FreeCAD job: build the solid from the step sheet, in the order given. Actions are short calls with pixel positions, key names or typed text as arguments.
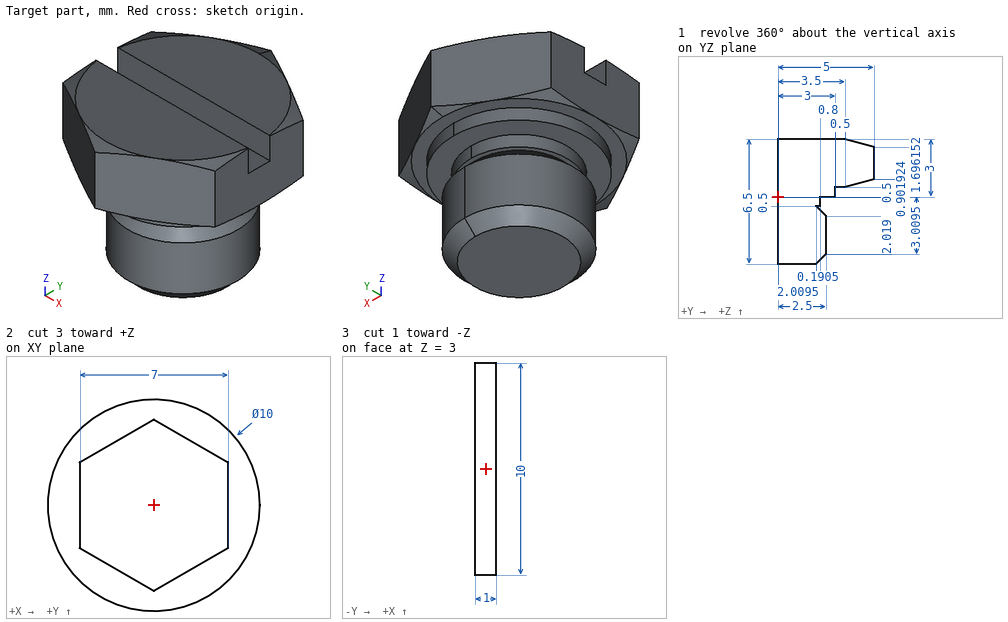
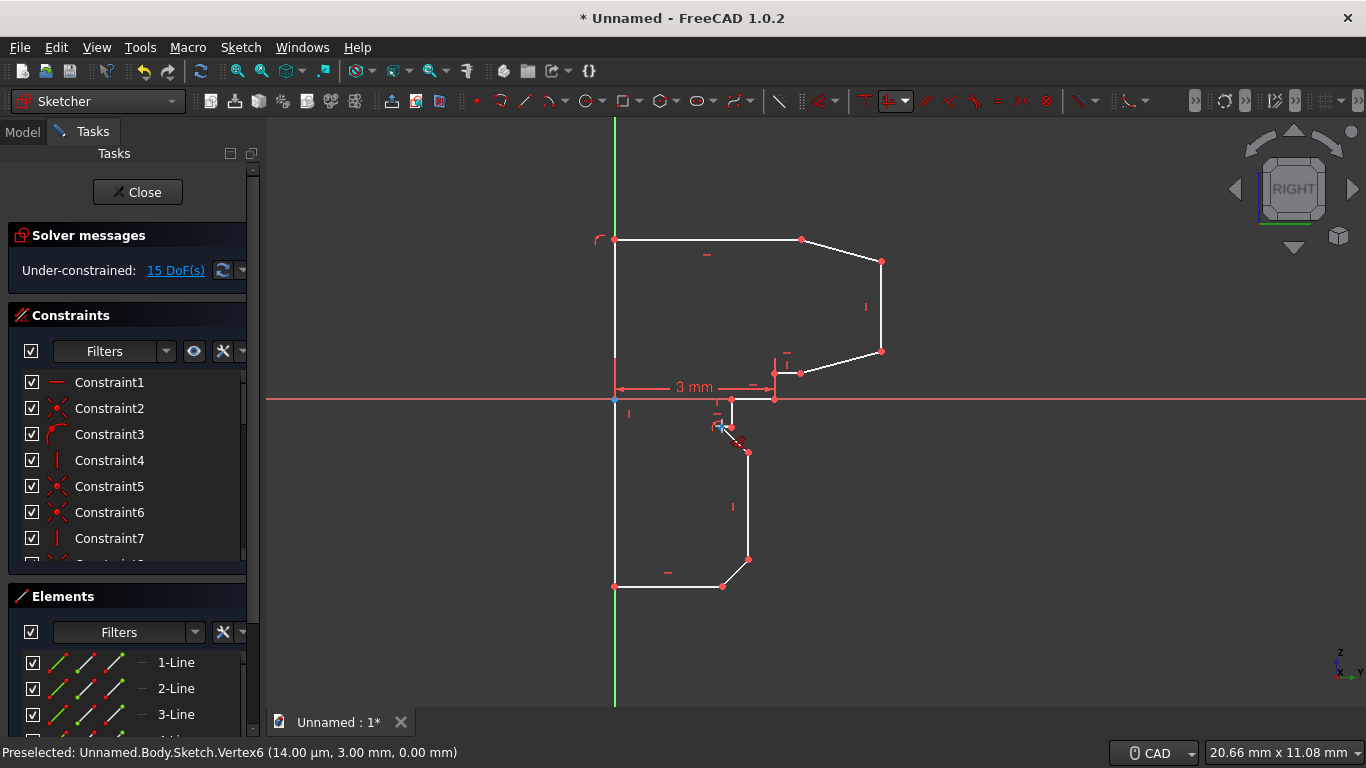
click(881, 352)
click(748, 318)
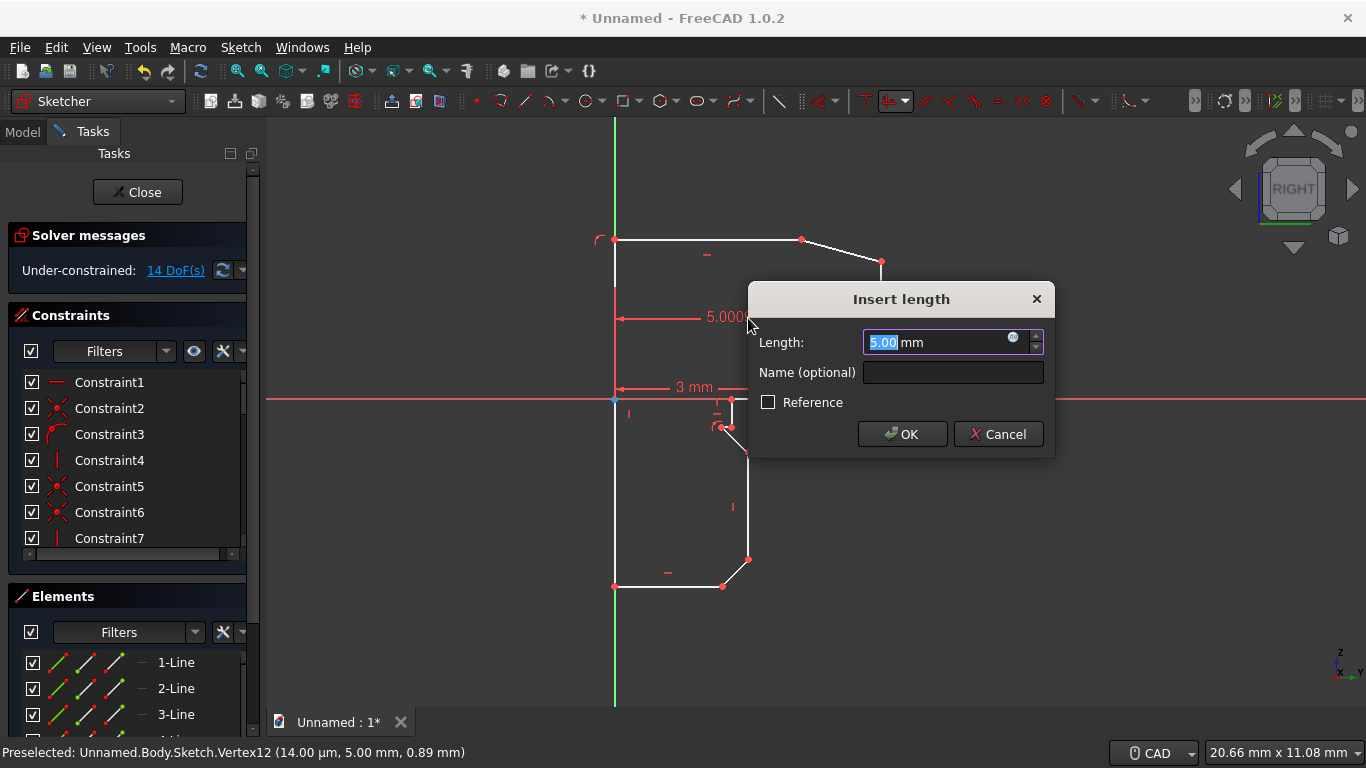
text(5)
key(Return)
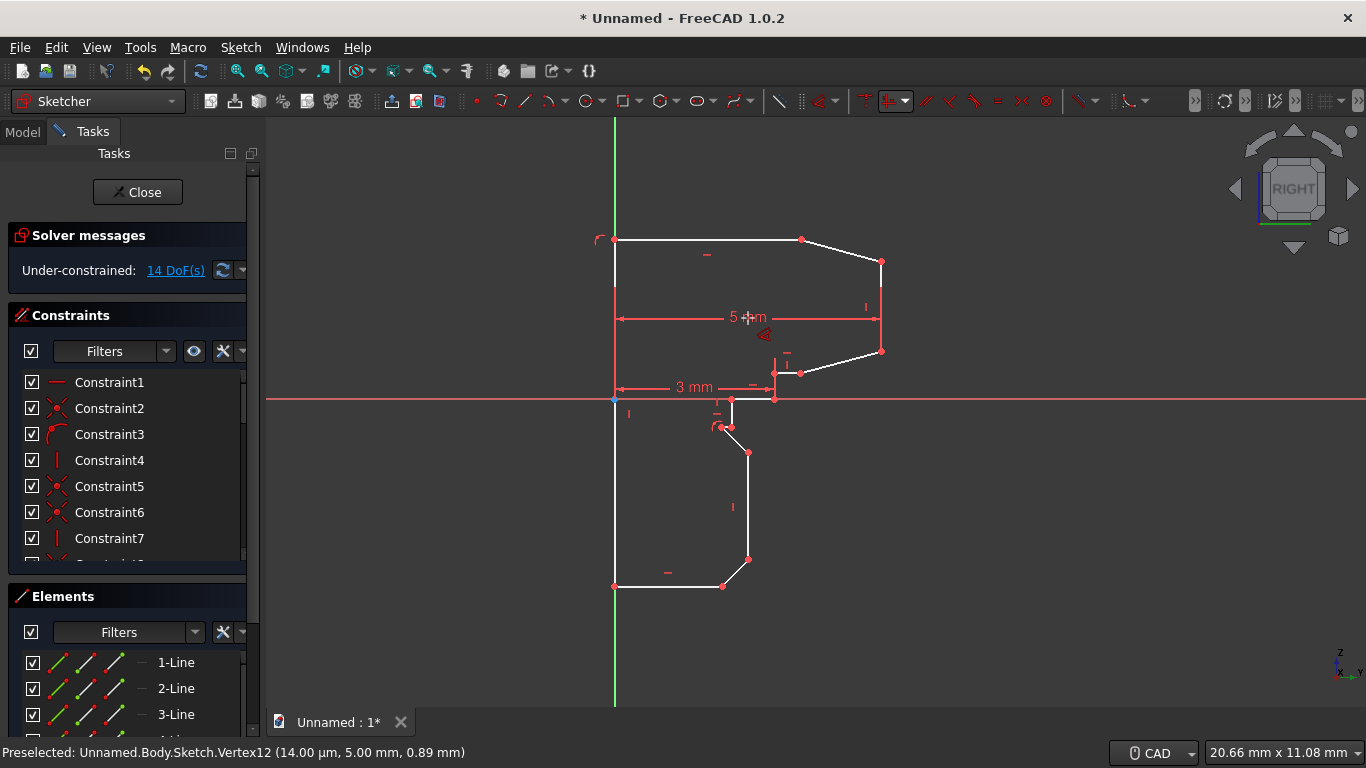
click(801, 240)
click(581, 320)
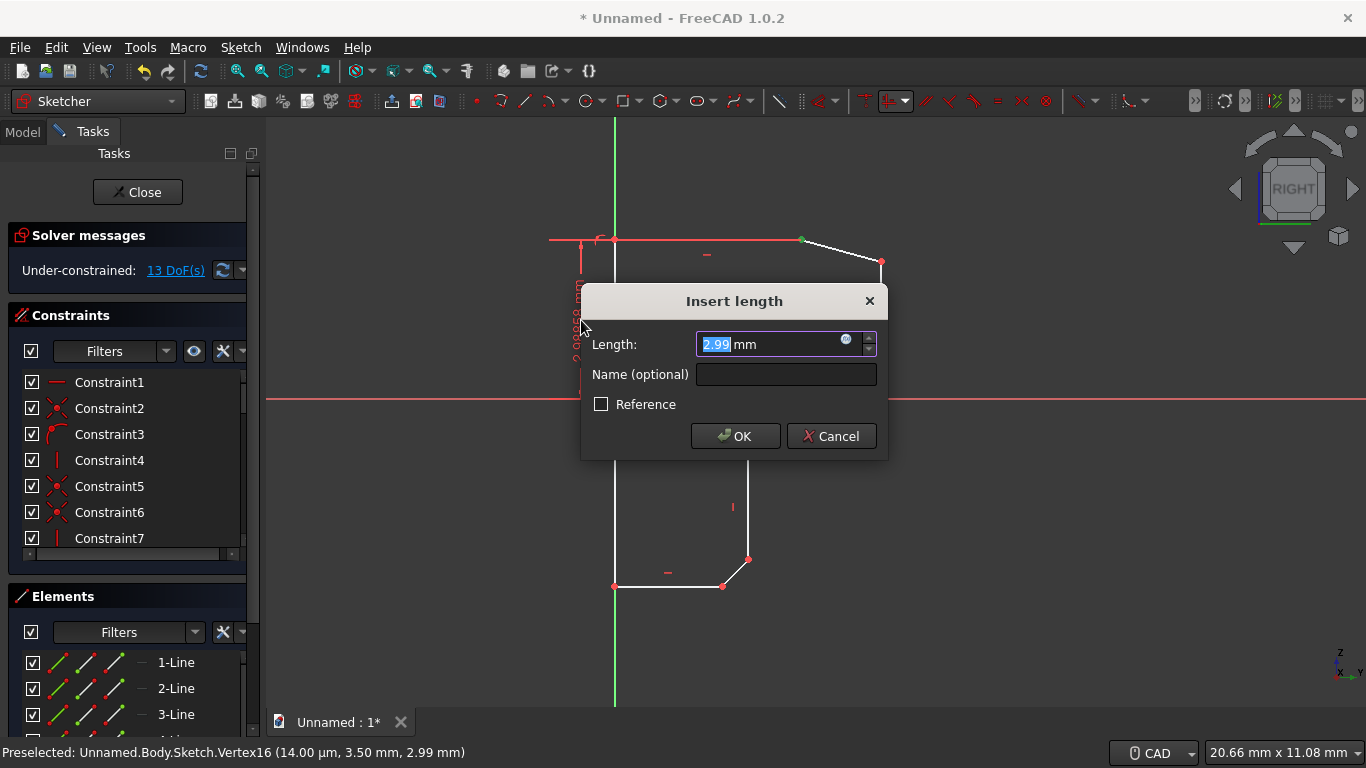
text(3)
key(Return)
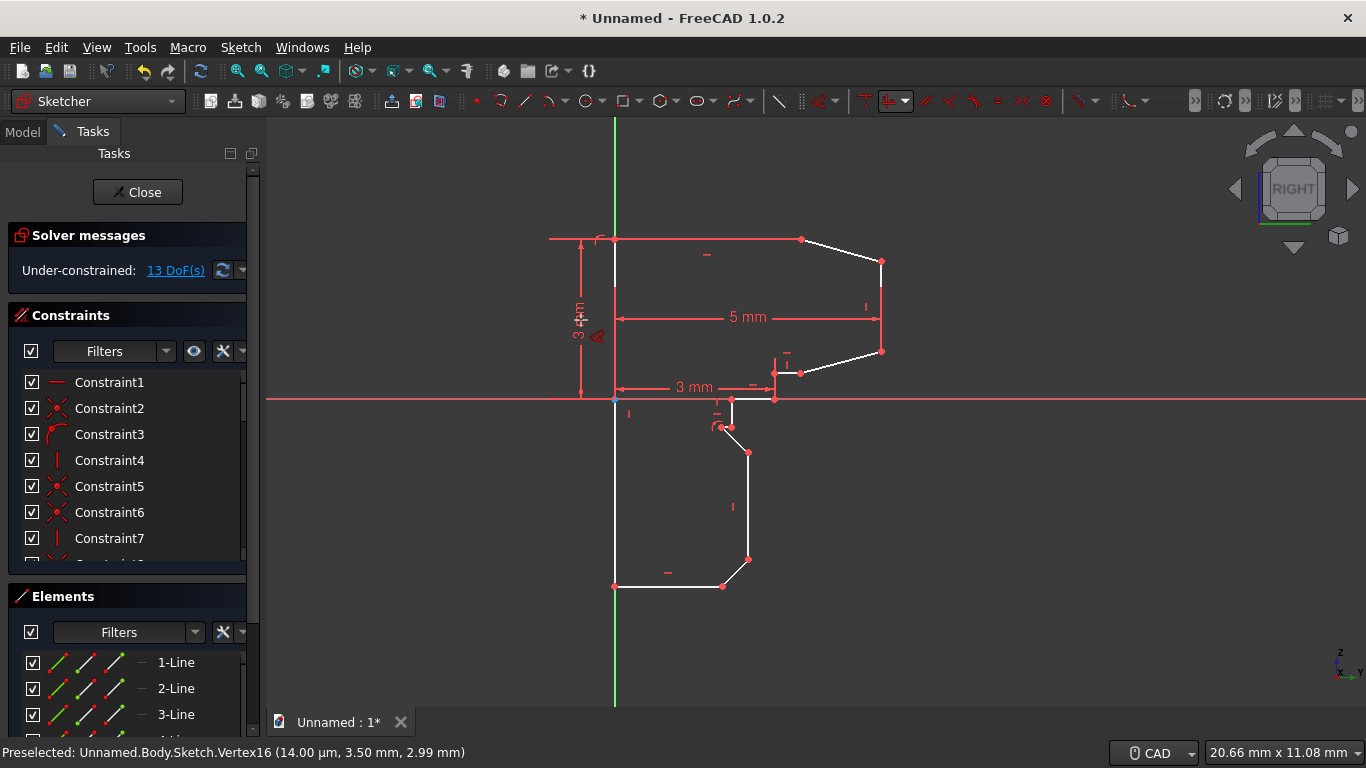
scroll(732, 416, up, 2)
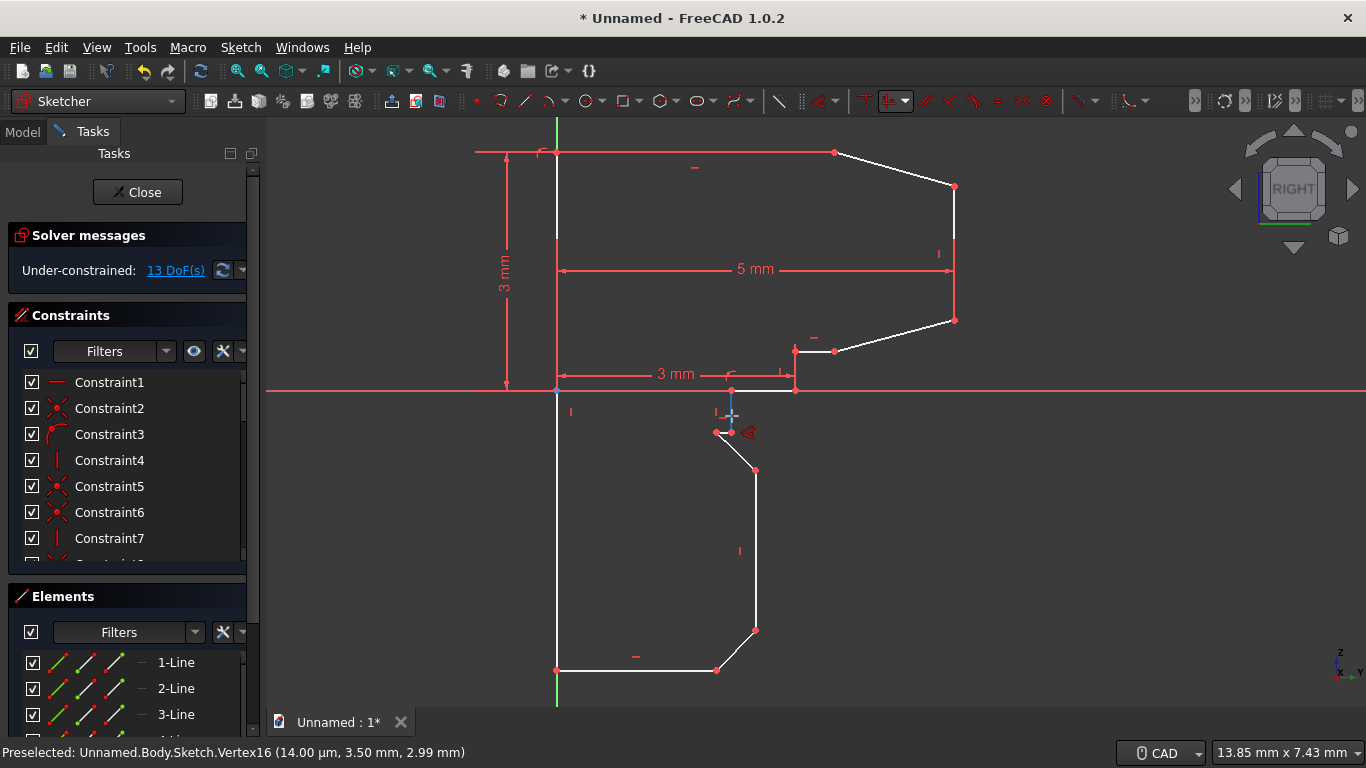
click(731, 416)
click(697, 412)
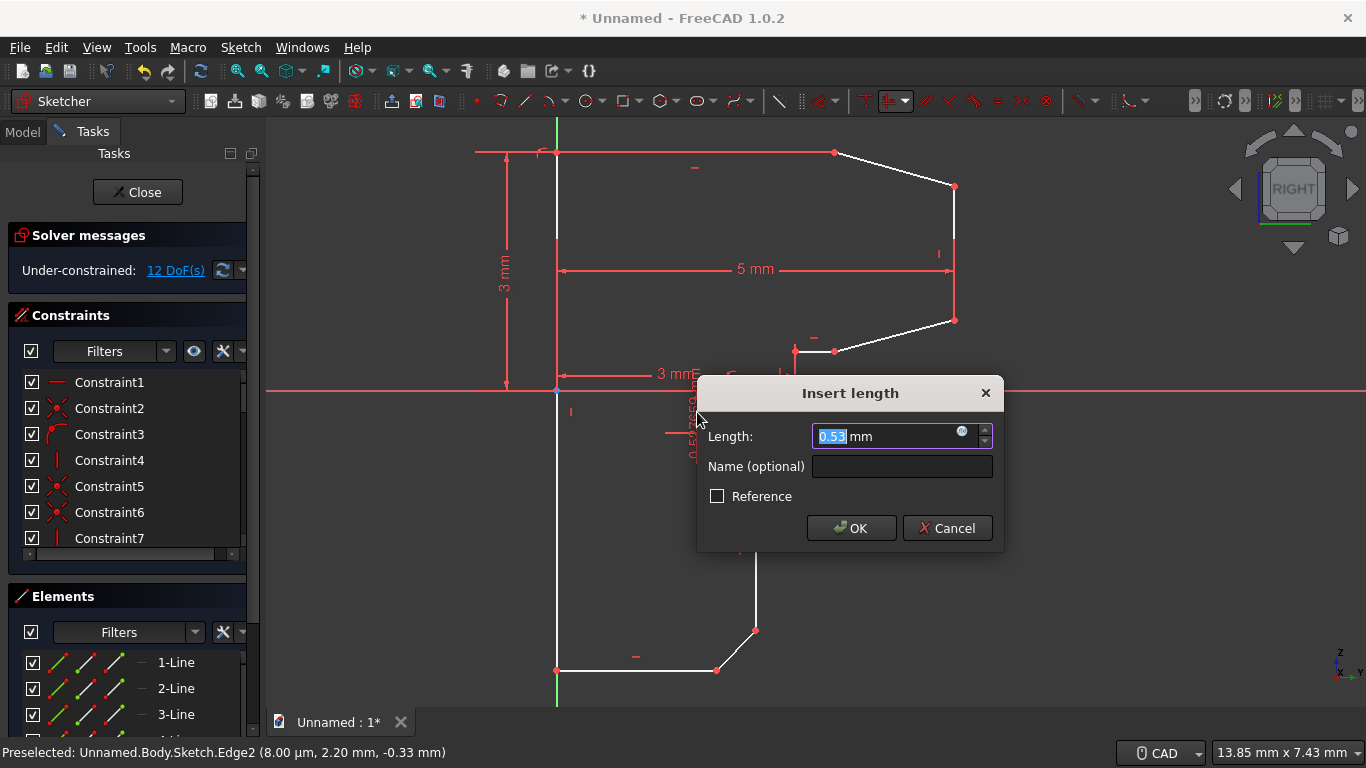
text(0.5)
key(Return)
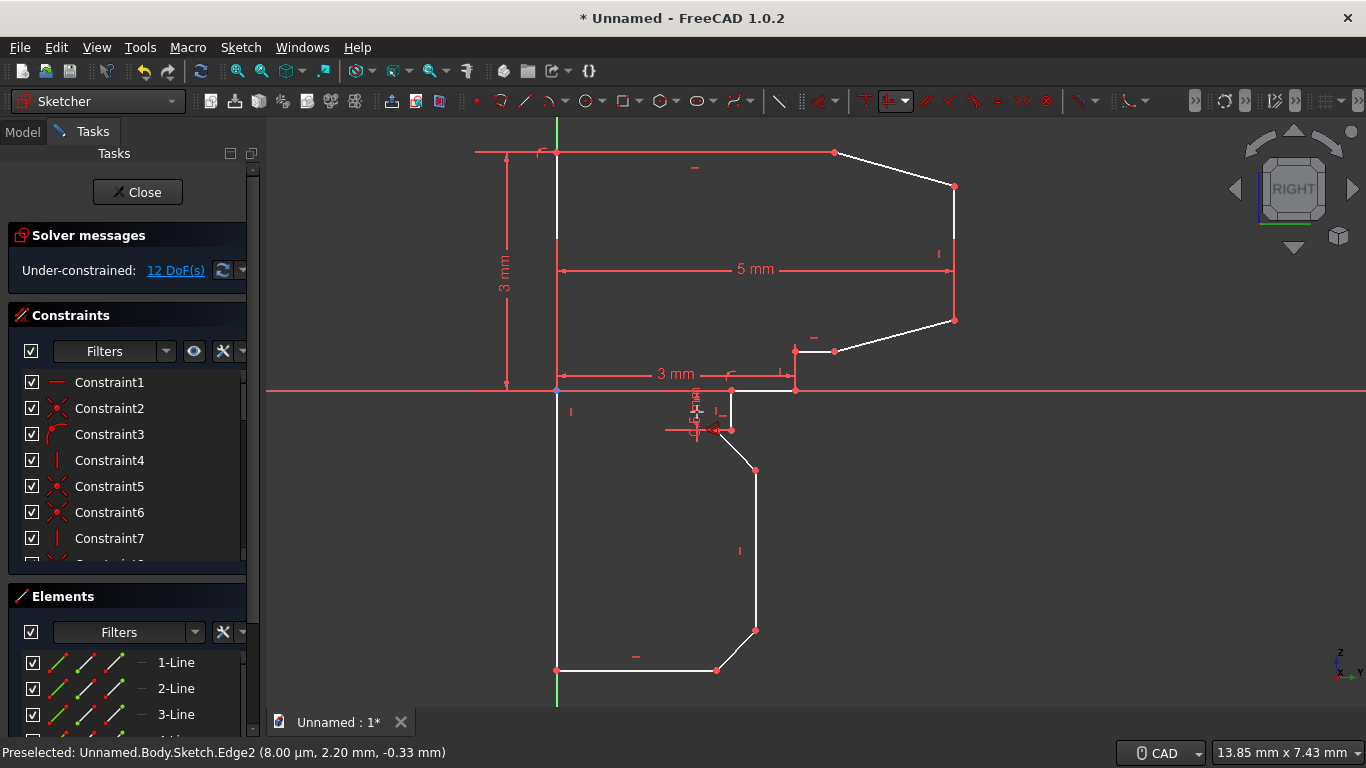
click(751, 391)
click(763, 357)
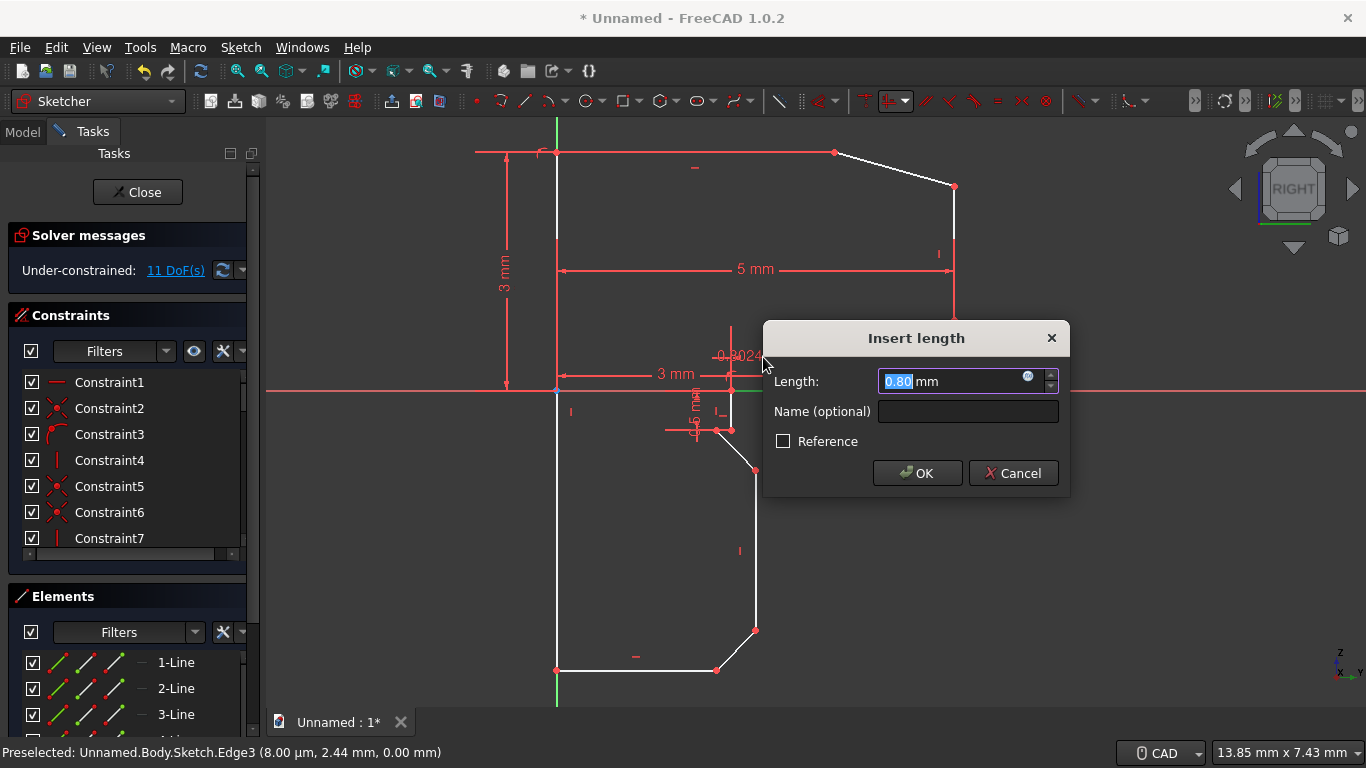
text(0.8)
key(Return)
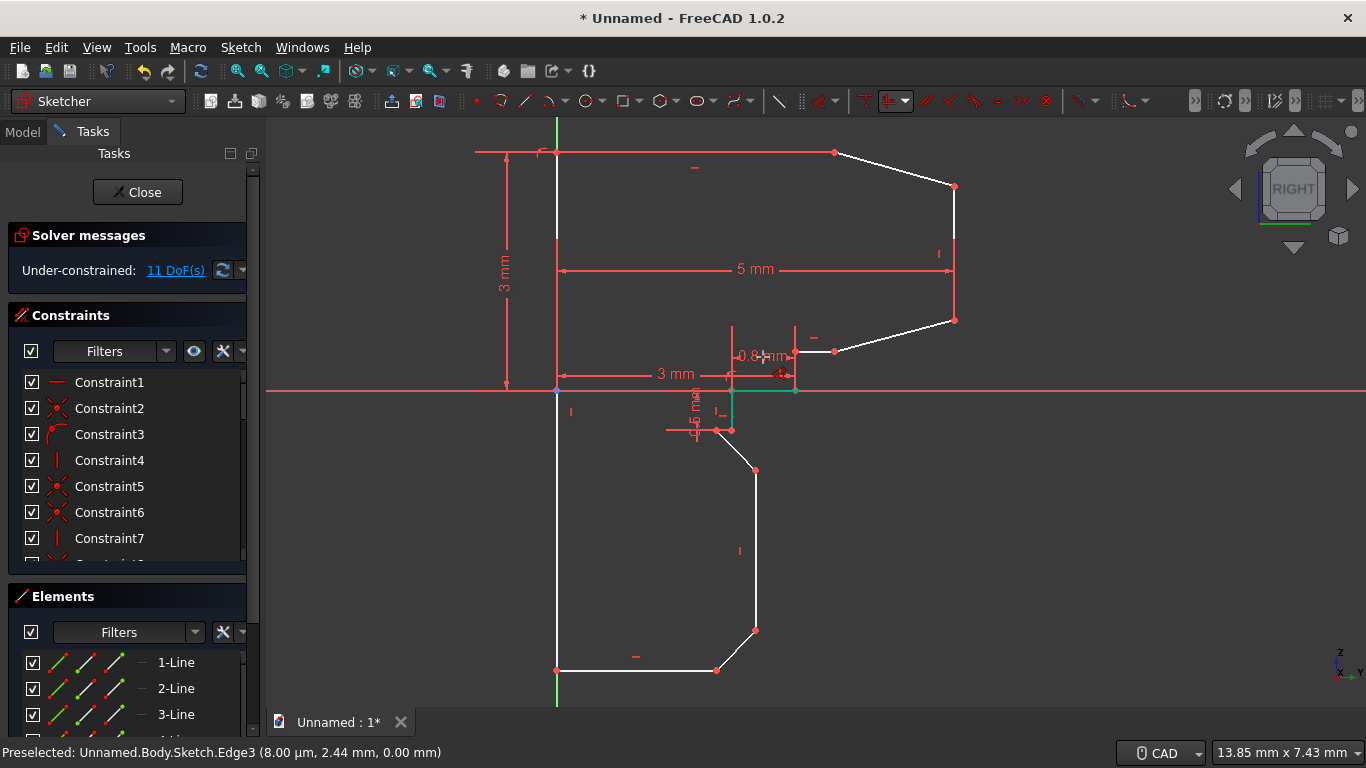
click(795, 379)
click(853, 371)